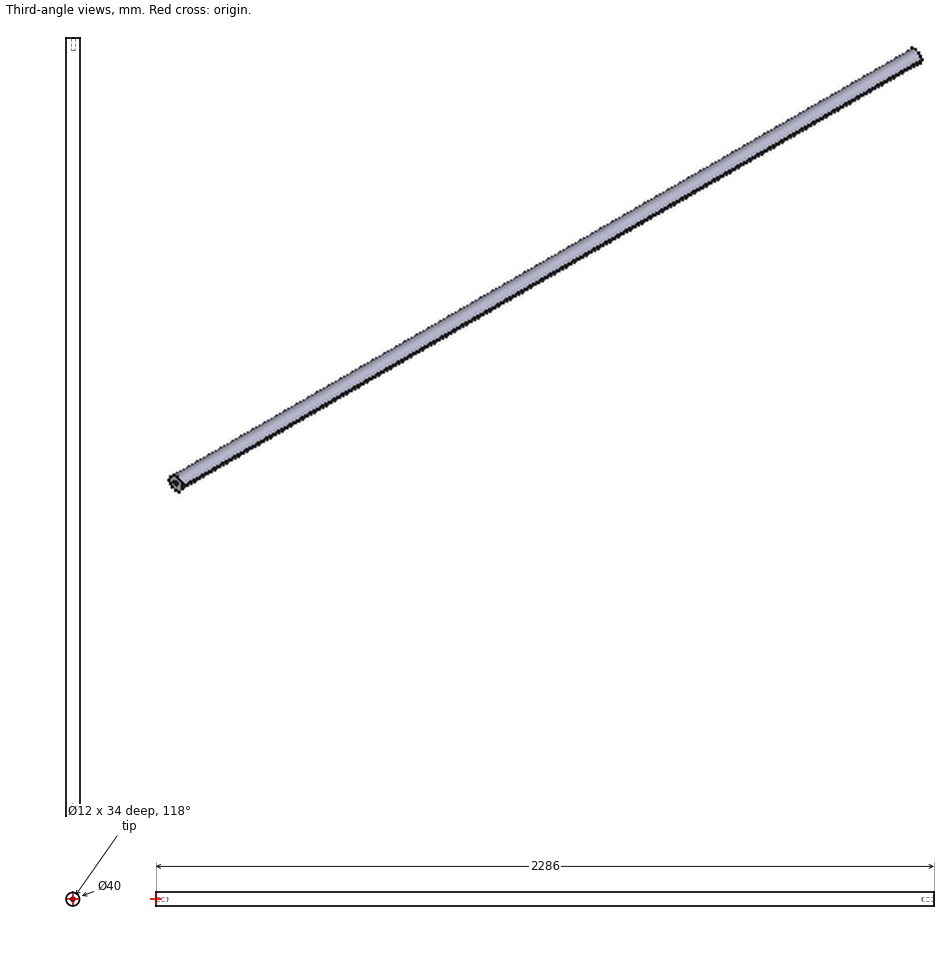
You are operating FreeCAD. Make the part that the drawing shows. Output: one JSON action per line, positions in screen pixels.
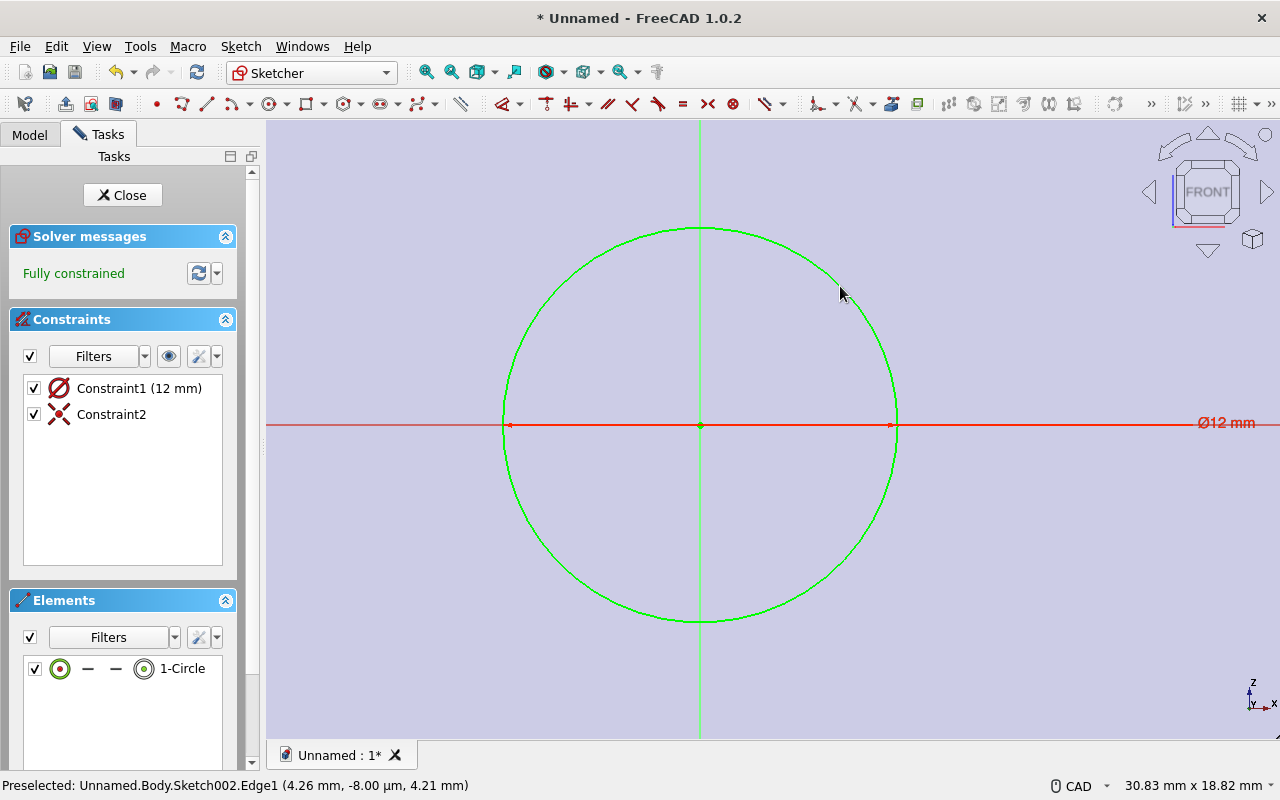
{"action": "left_click", "coordinate": [123, 195]}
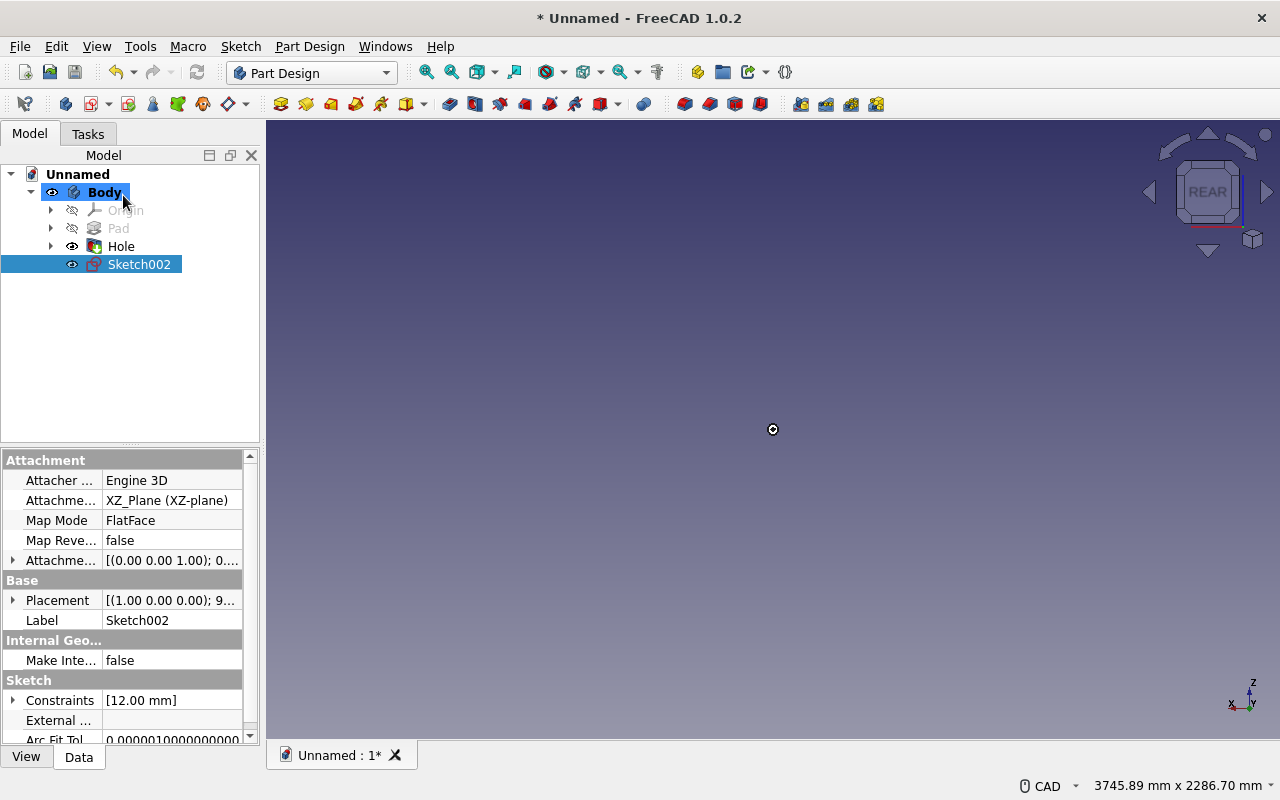
{"action": "left_click", "coordinate": [475, 104]}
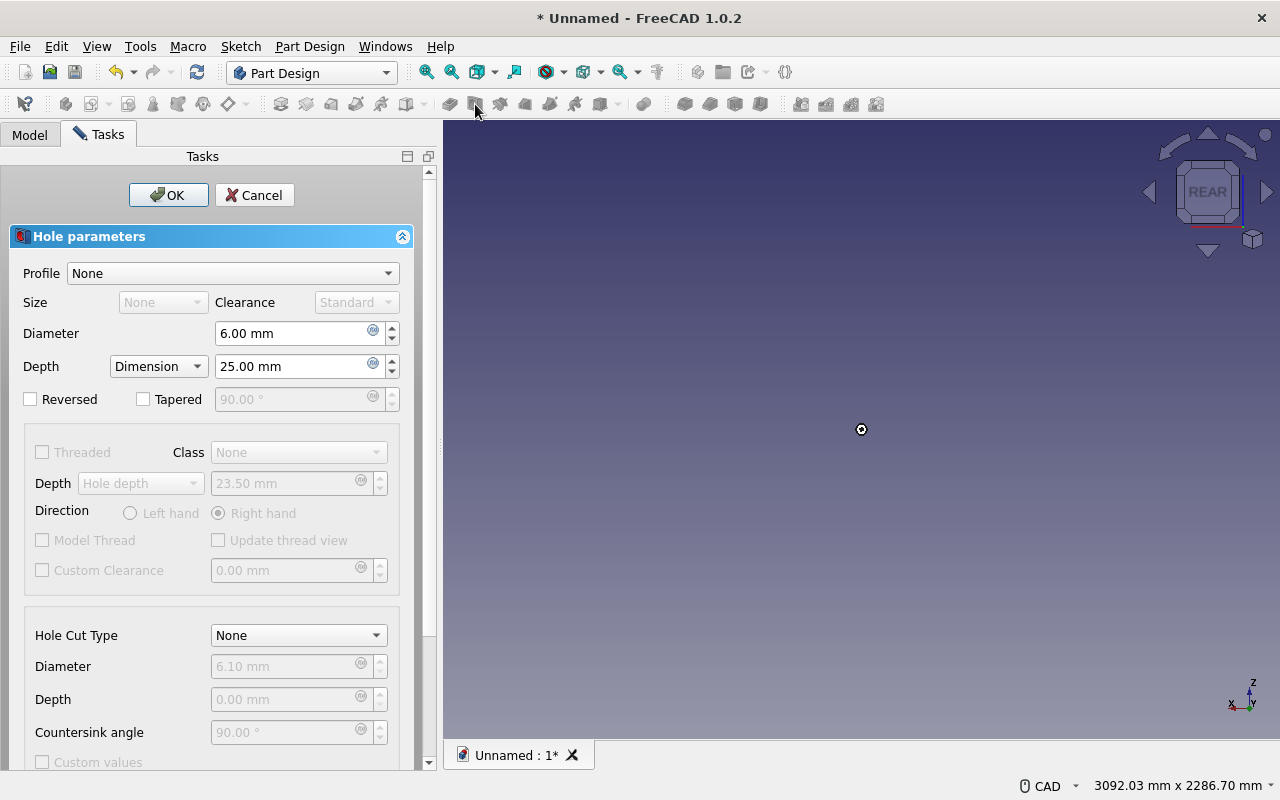
{"action": "triple_click", "coordinate": [300, 334]}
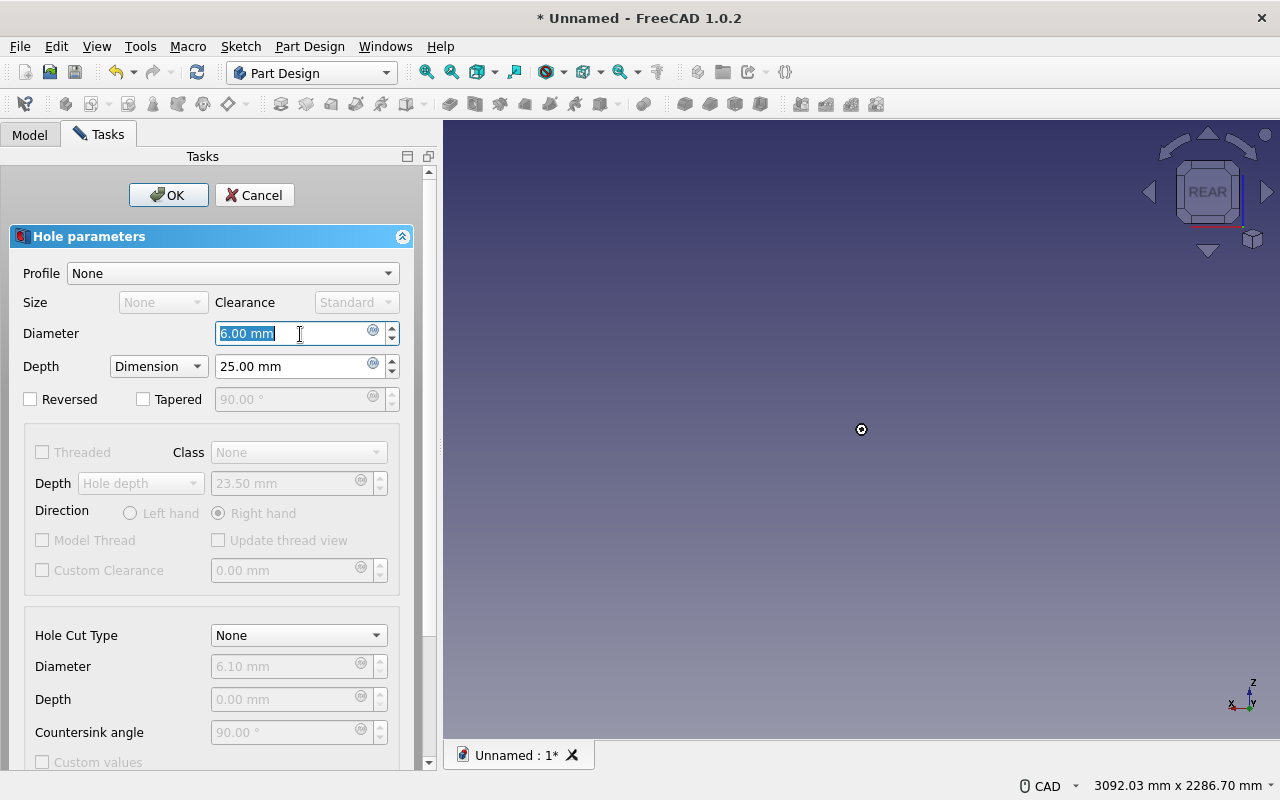
{"action": "type", "text": "12"}
{"action": "key", "text": "Tab"}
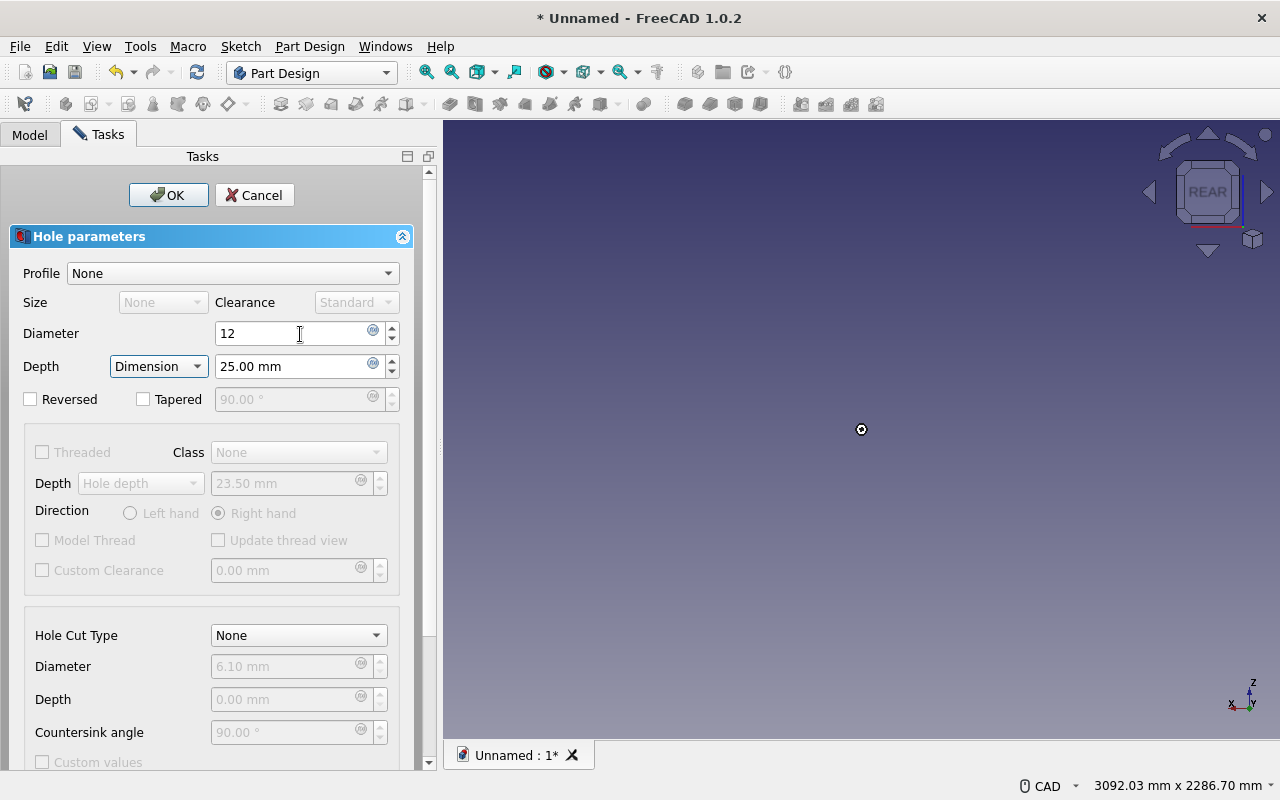
{"action": "triple_click", "coordinate": [300, 366]}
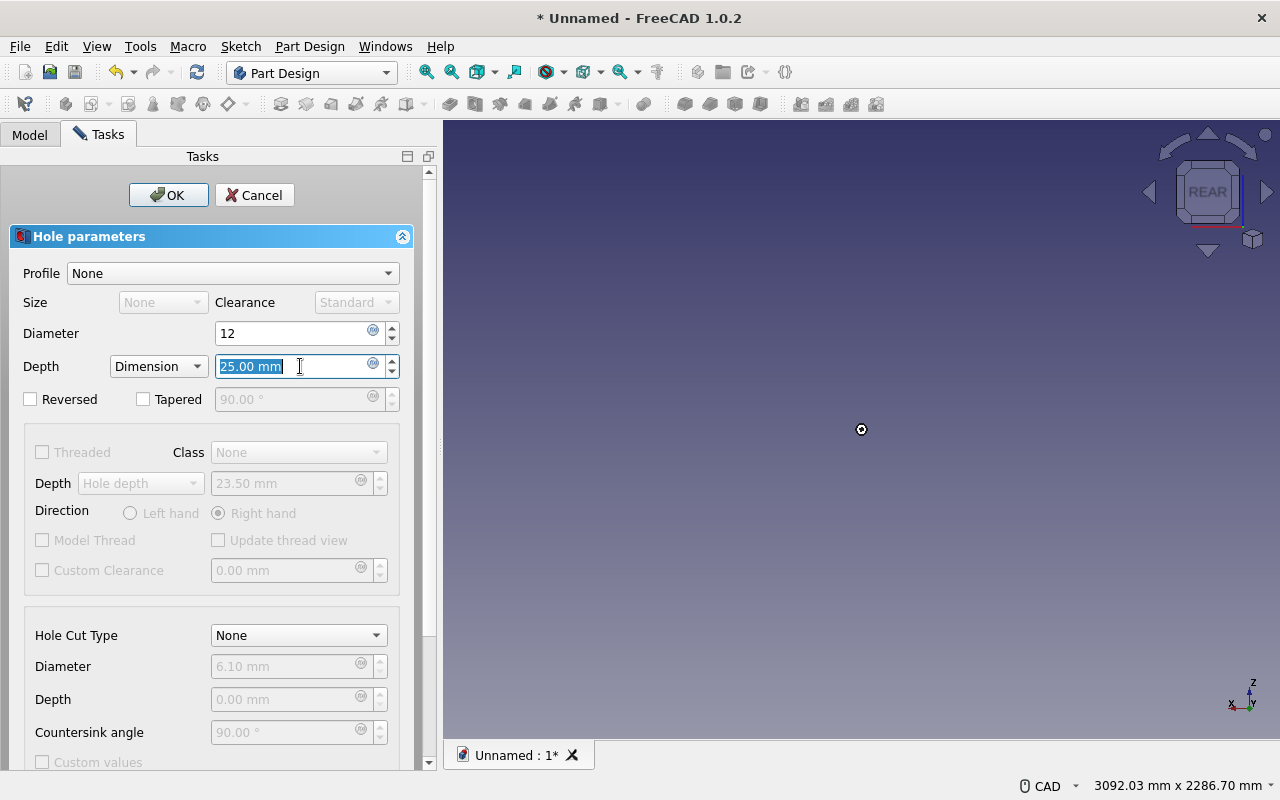
{"action": "type", "text": "34"}
{"action": "key", "text": "Tab"}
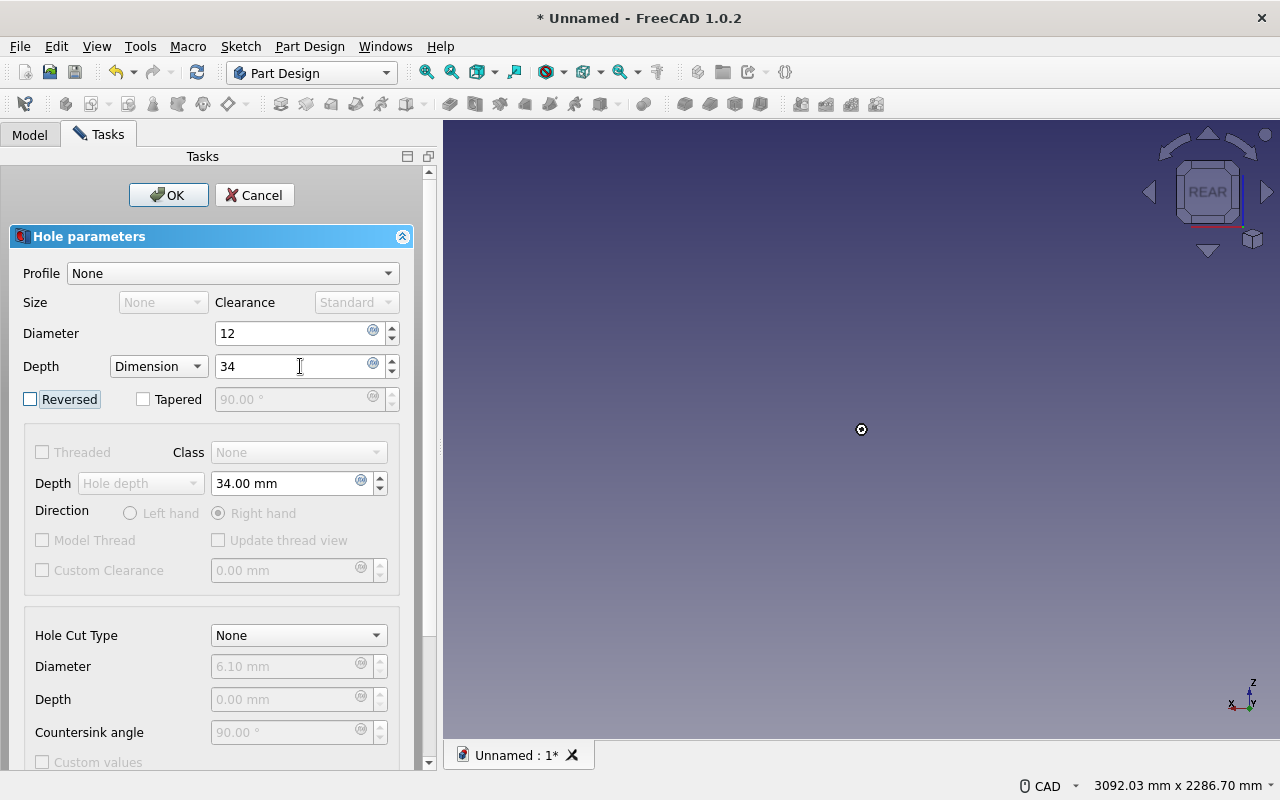
{"action": "left_click", "coordinate": [169, 195]}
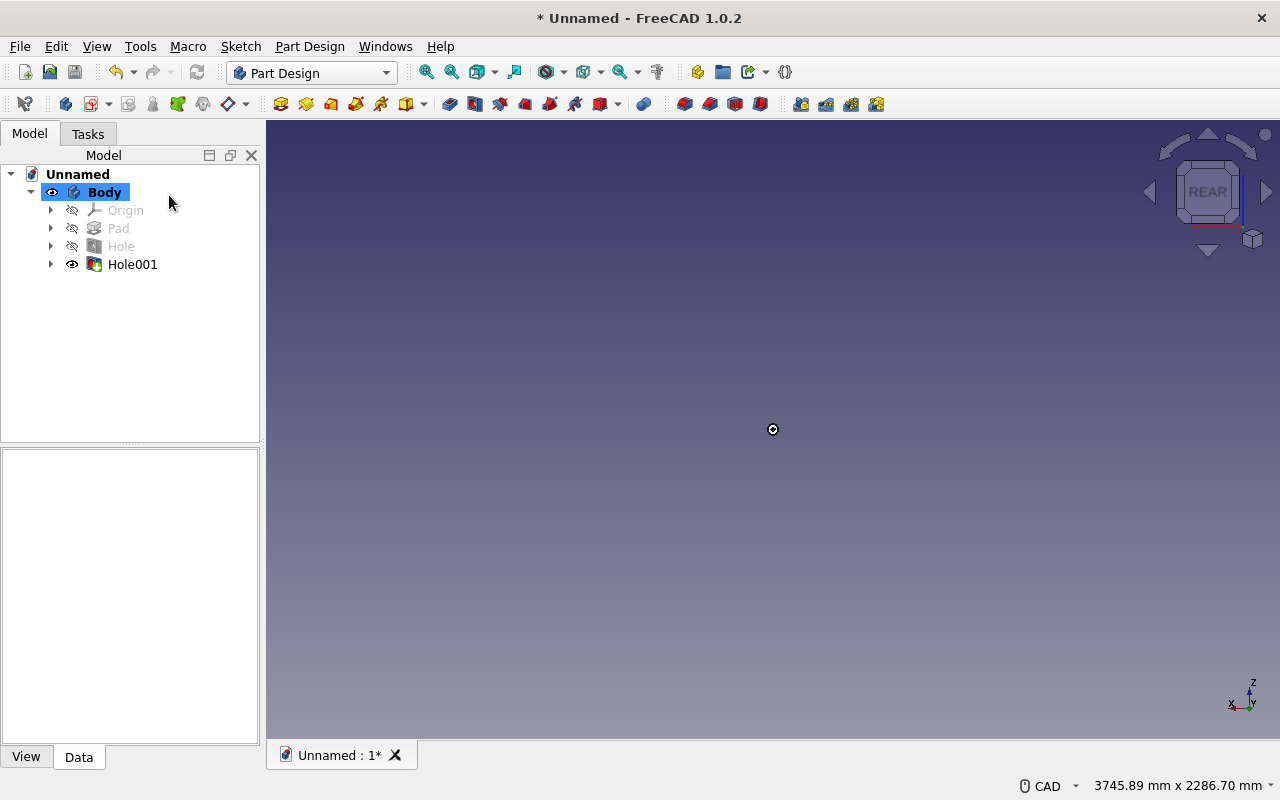
{"action": "key", "text": "0"}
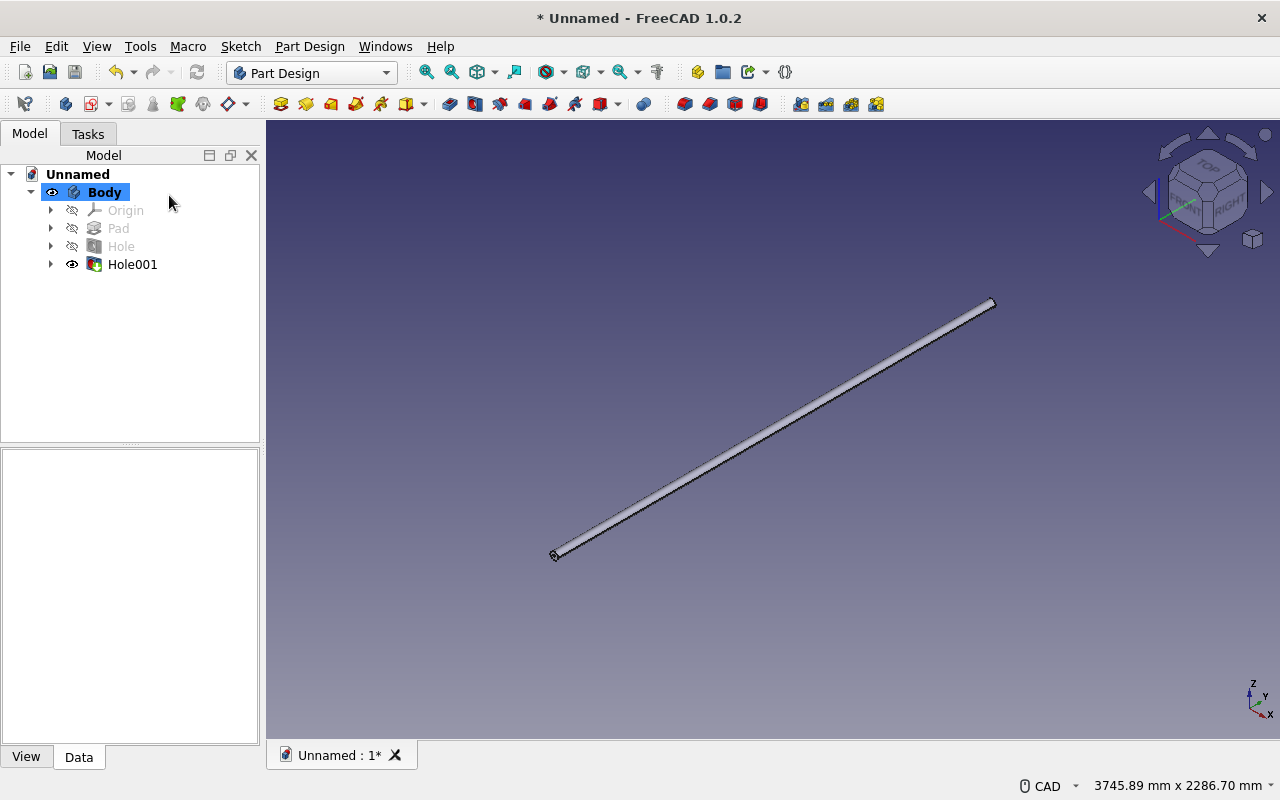
{"action": "left_click", "coordinate": [427, 72]}